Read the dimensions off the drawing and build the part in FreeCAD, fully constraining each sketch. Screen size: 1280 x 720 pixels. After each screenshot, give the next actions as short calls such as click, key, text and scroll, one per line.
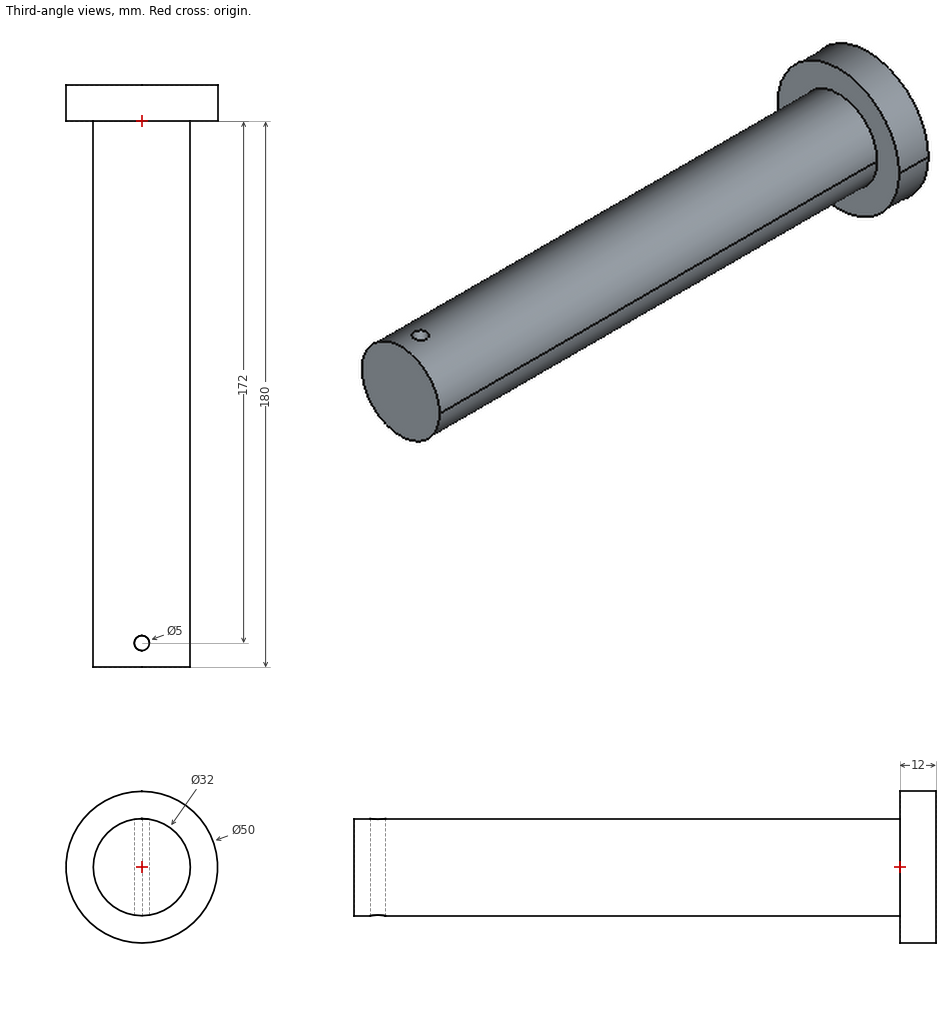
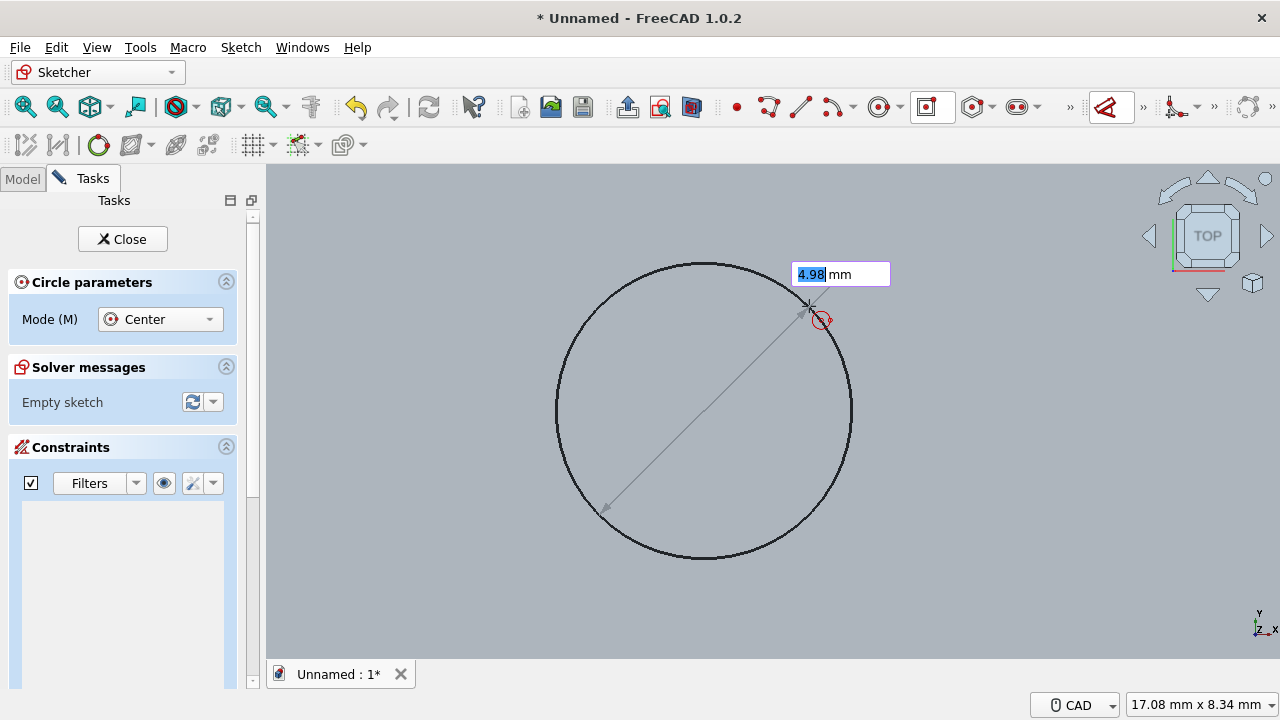
text(5)
key(Return)
key(Escape)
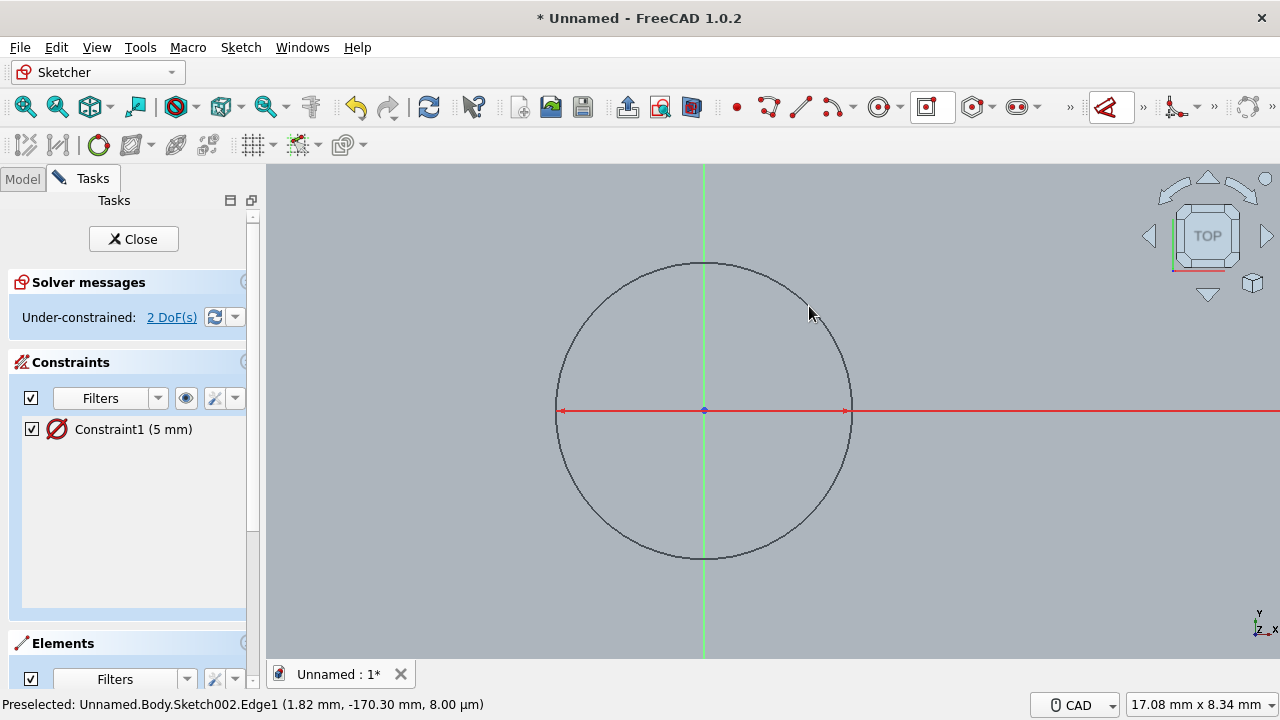
click(704, 411)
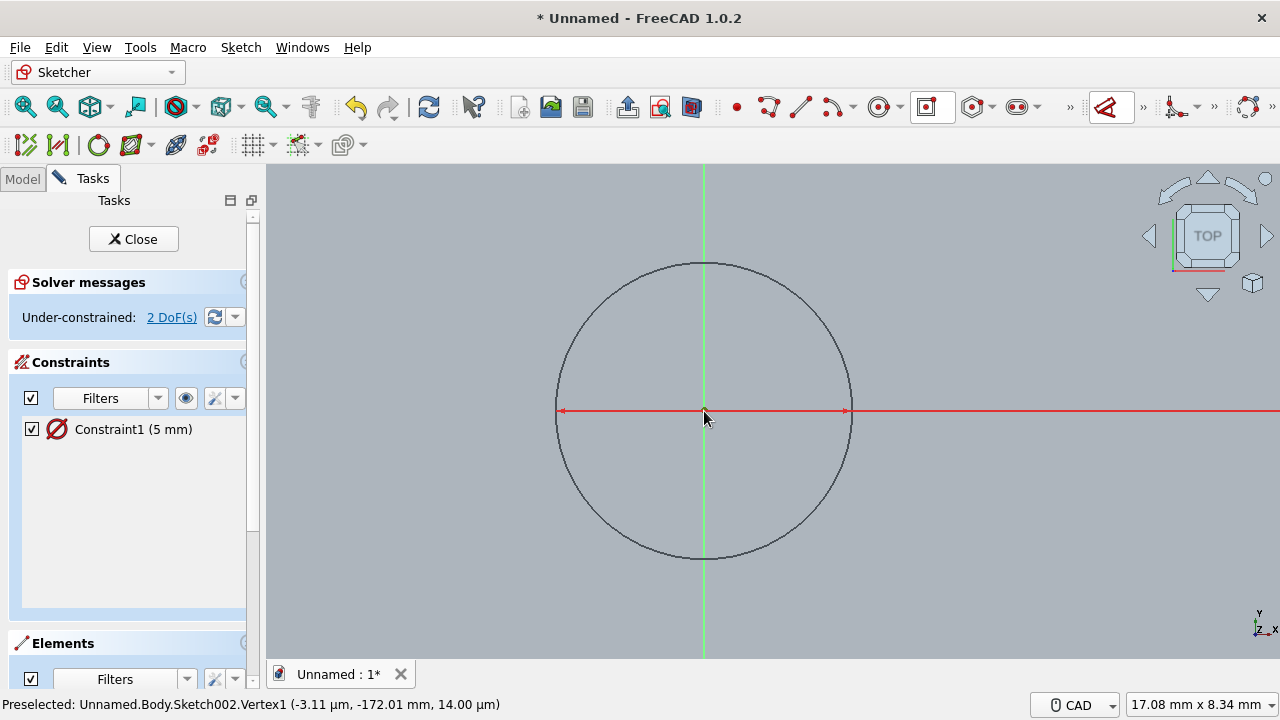
click(704, 600)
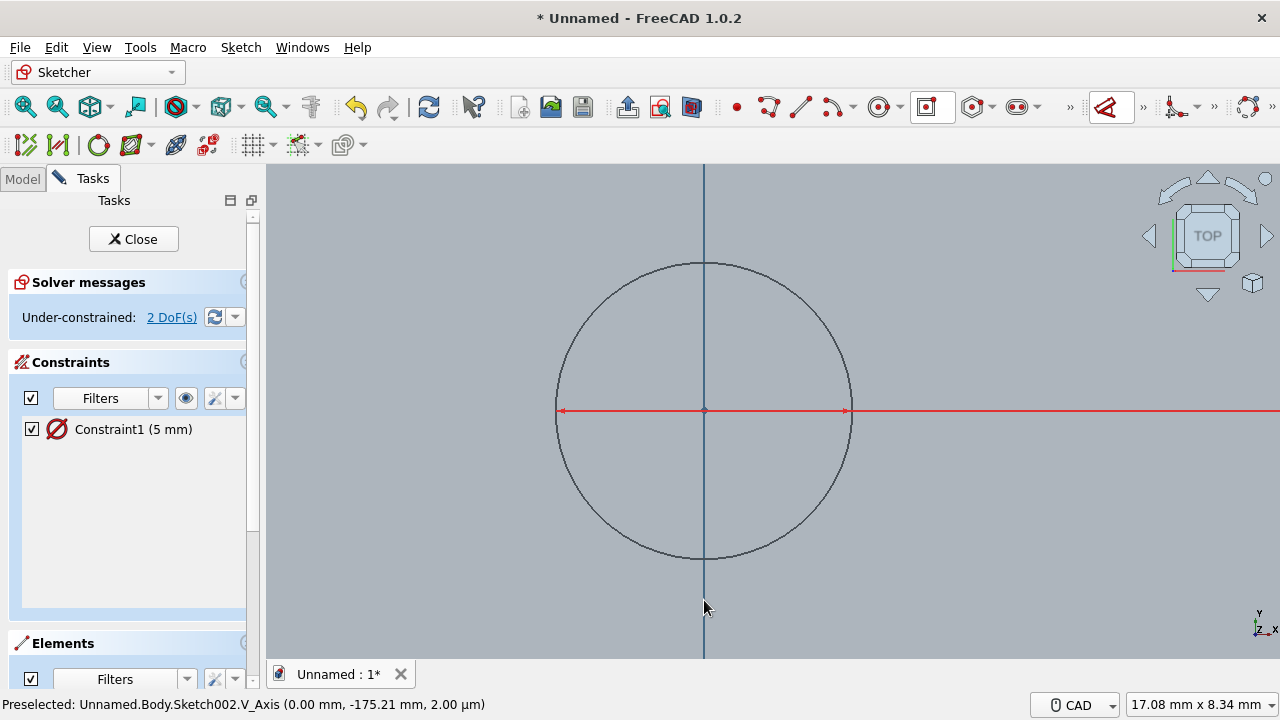
key(c)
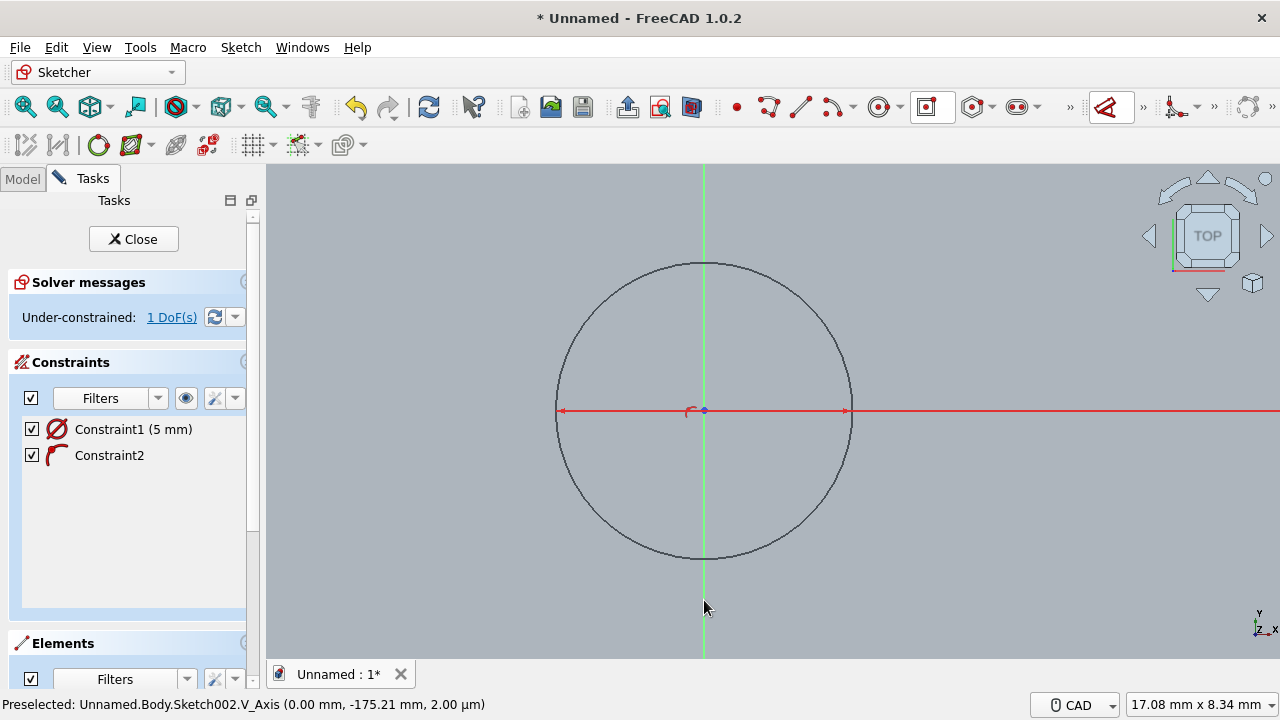
click(1106, 108)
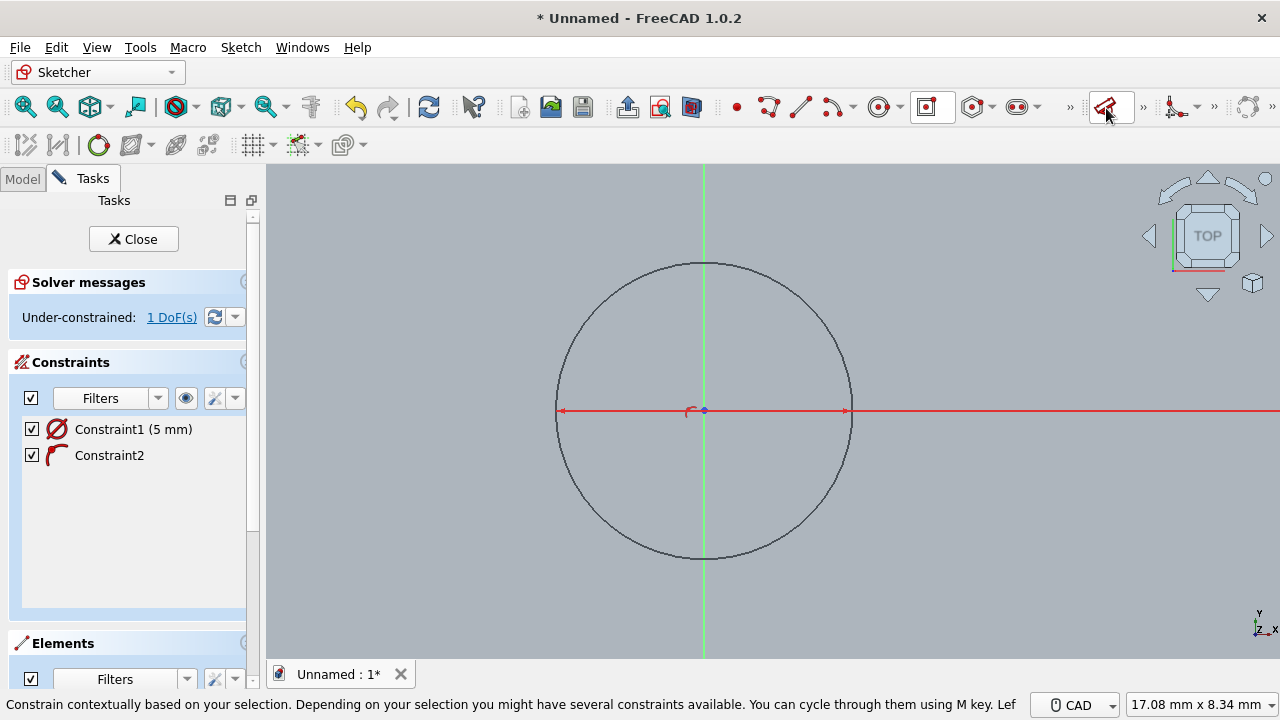
click(704, 411)
click(738, 302)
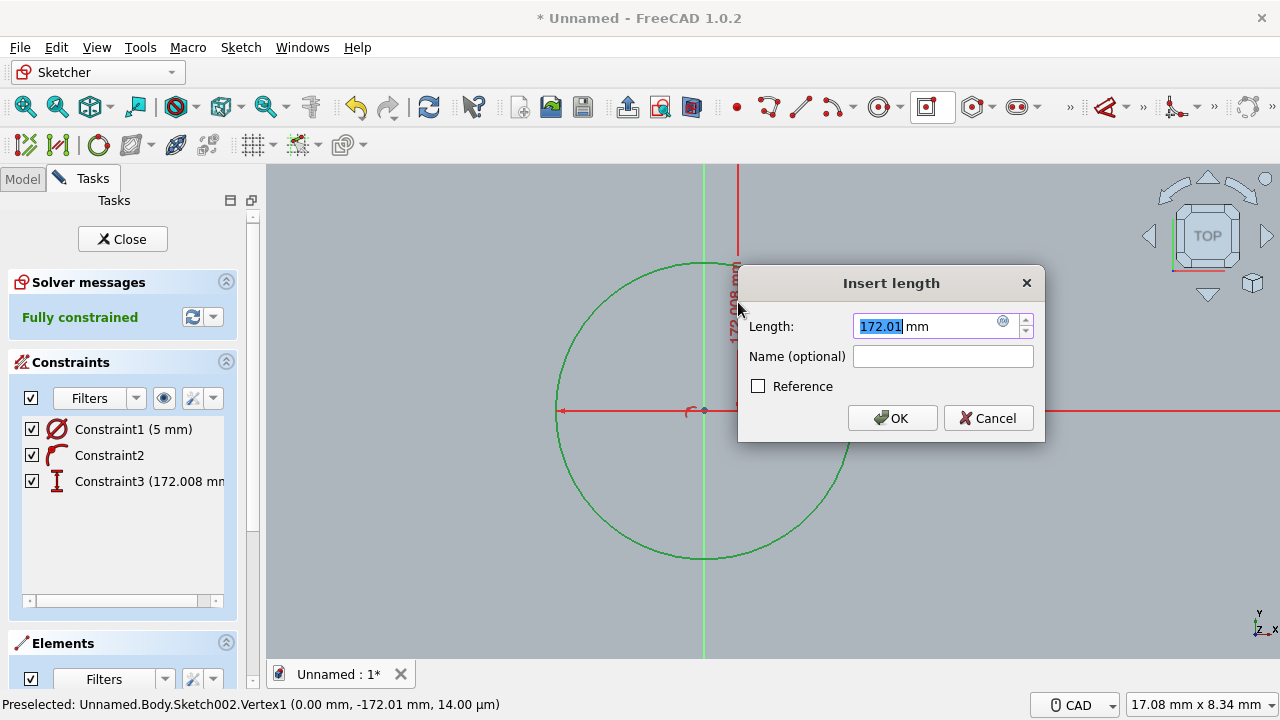
text(172)
key(Return)
key(Escape)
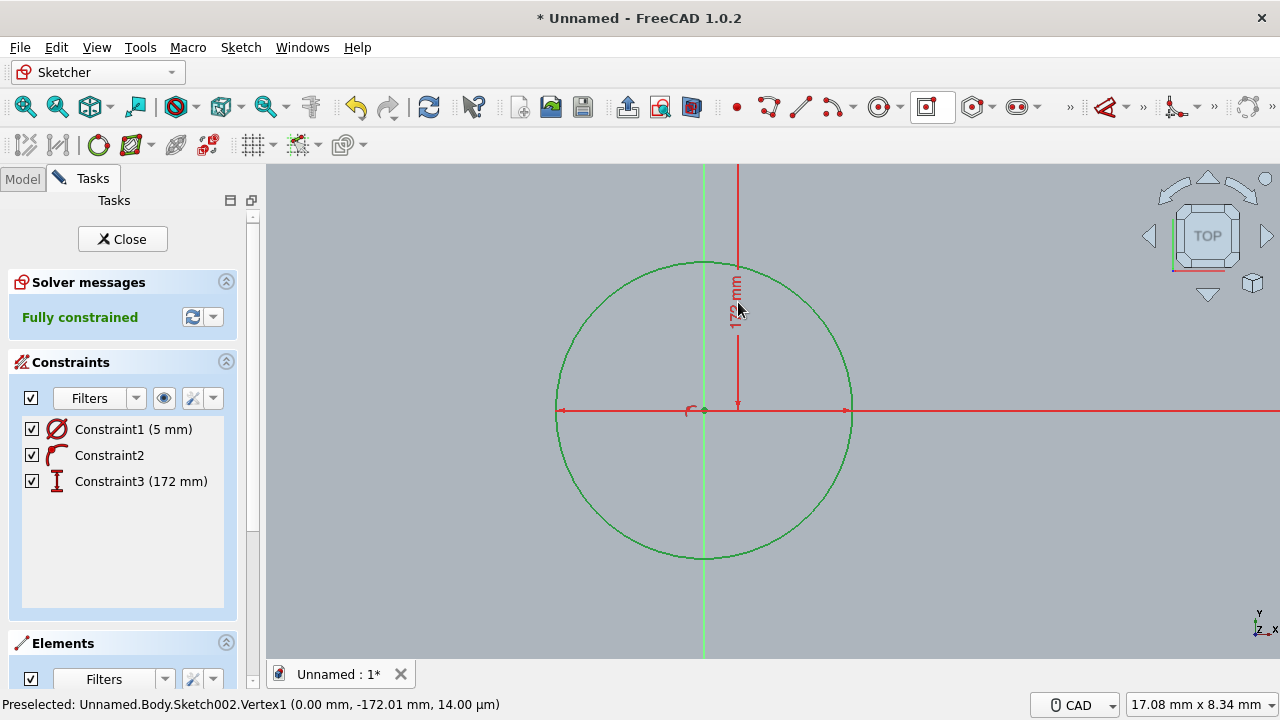
click(123, 239)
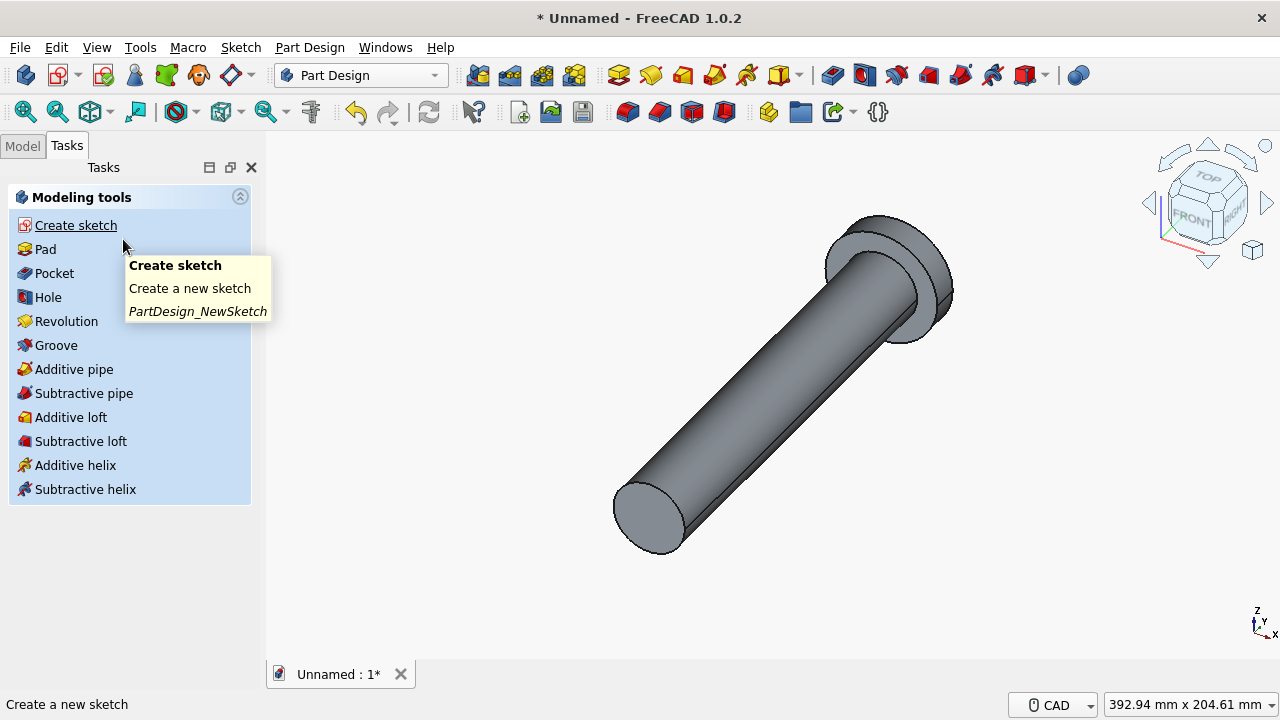
click(834, 76)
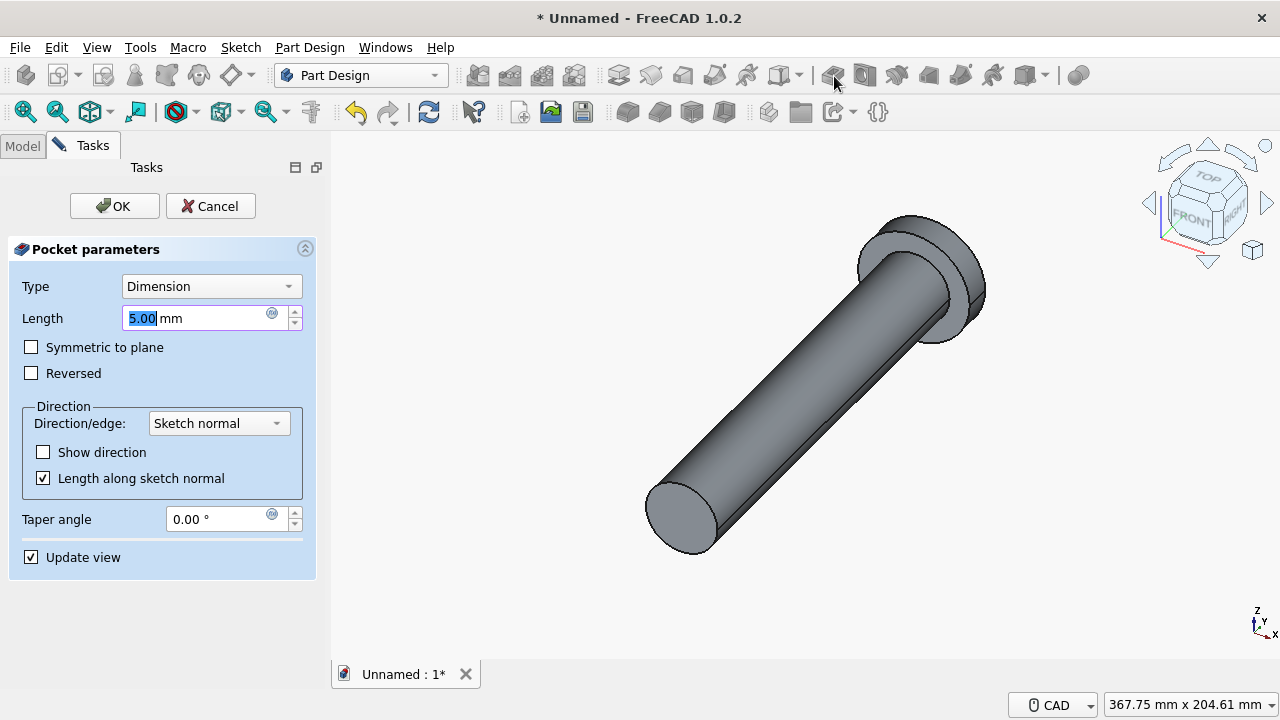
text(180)
key(Tab)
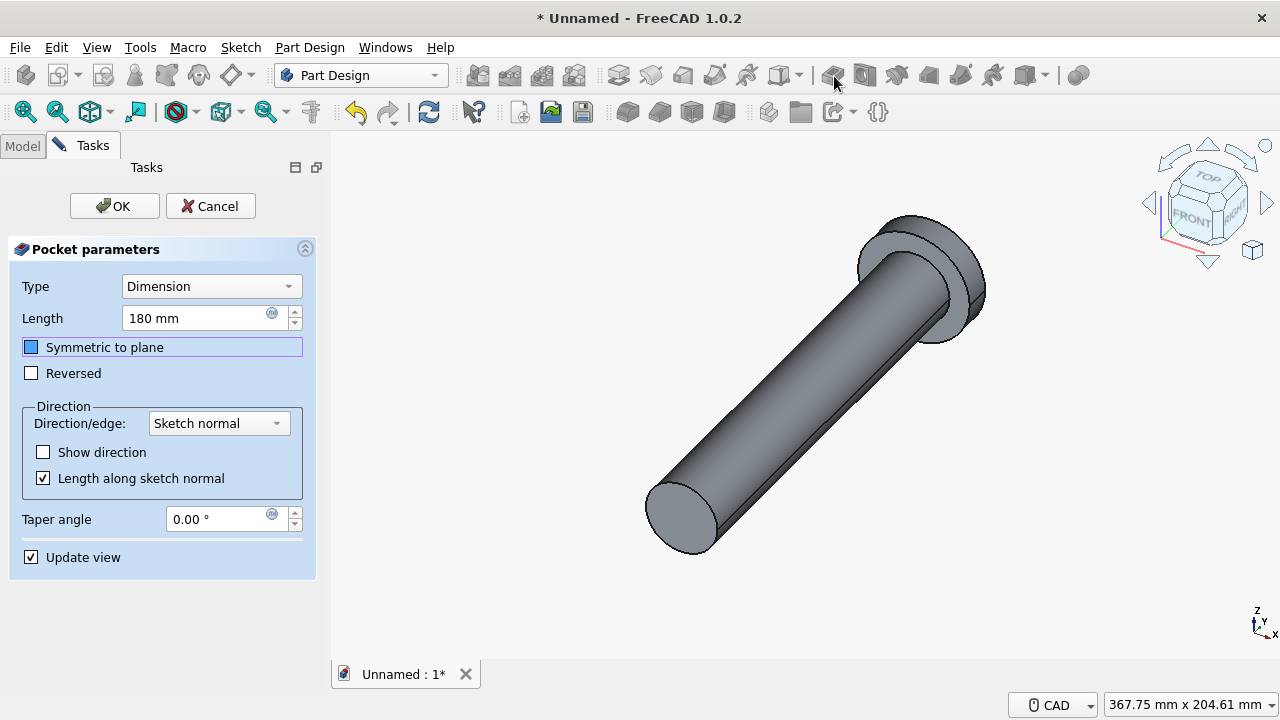
click(30, 347)